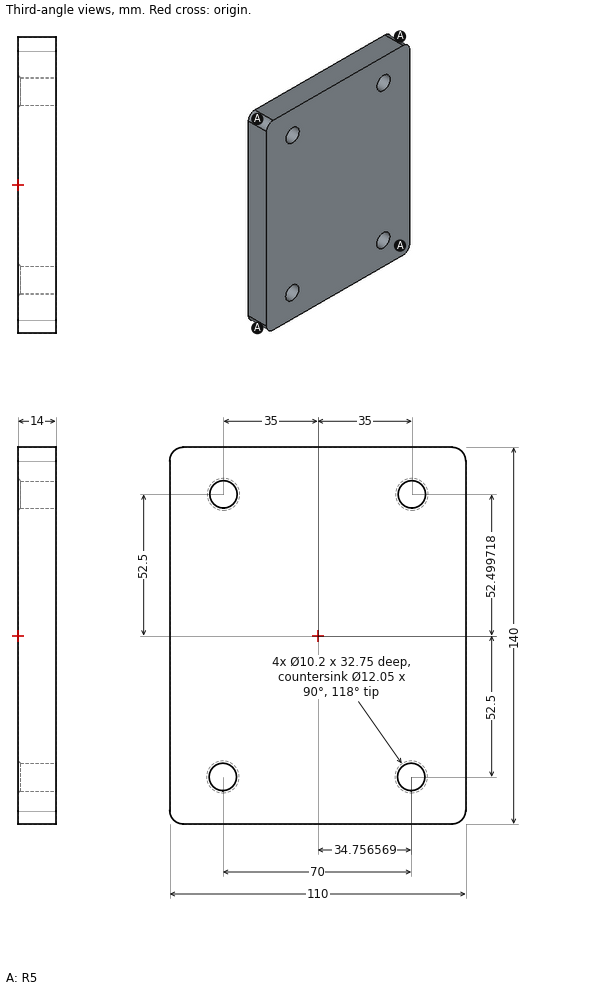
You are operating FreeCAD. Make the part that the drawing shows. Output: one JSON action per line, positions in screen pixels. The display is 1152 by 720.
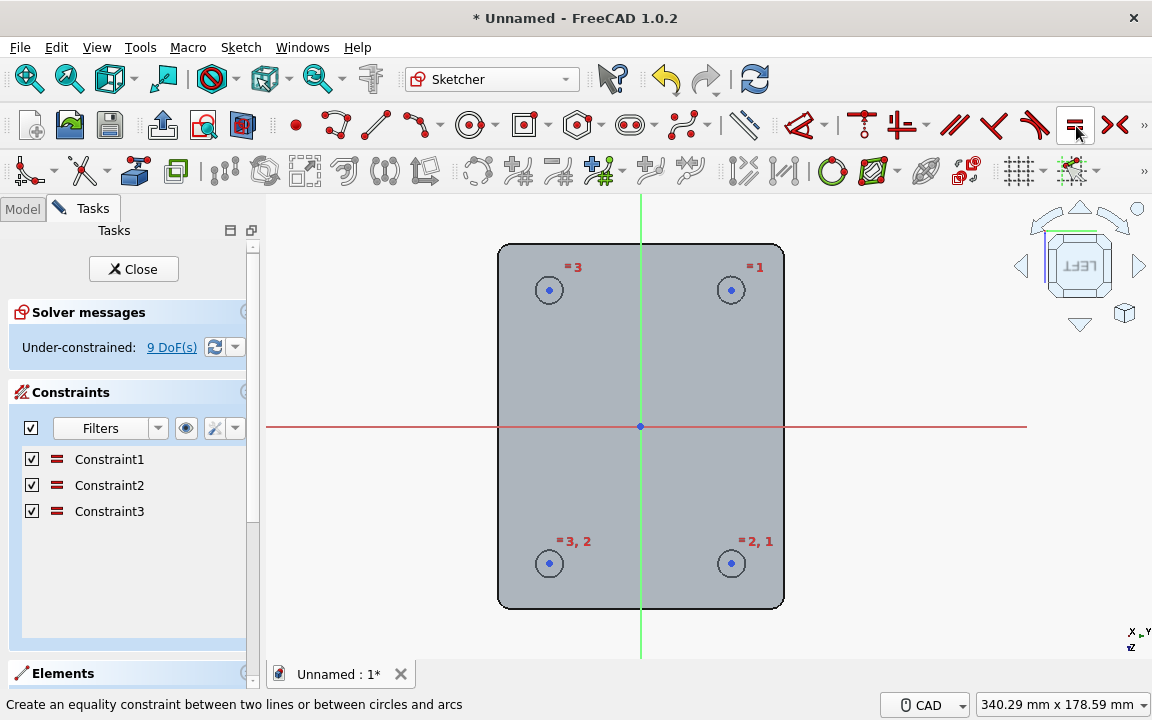
{"action": "left_click", "coordinate": [800, 126]}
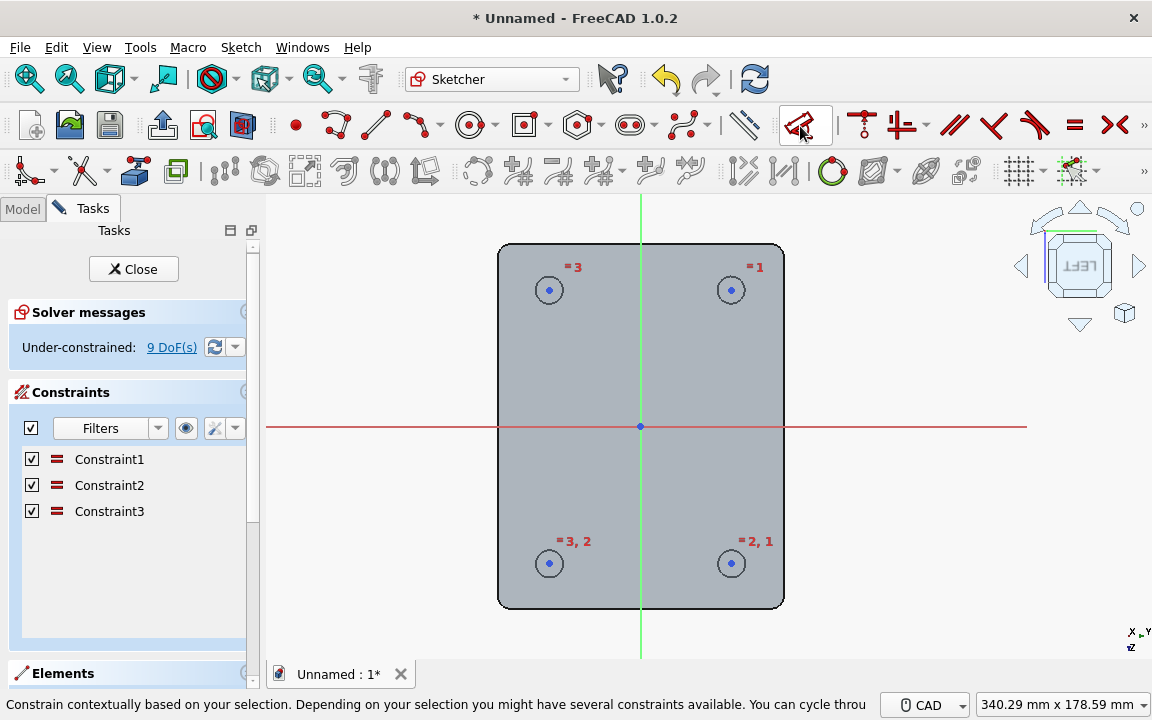
{"action": "scroll", "coordinate": [741, 280], "scroll_direction": "up", "scroll_amount": 3}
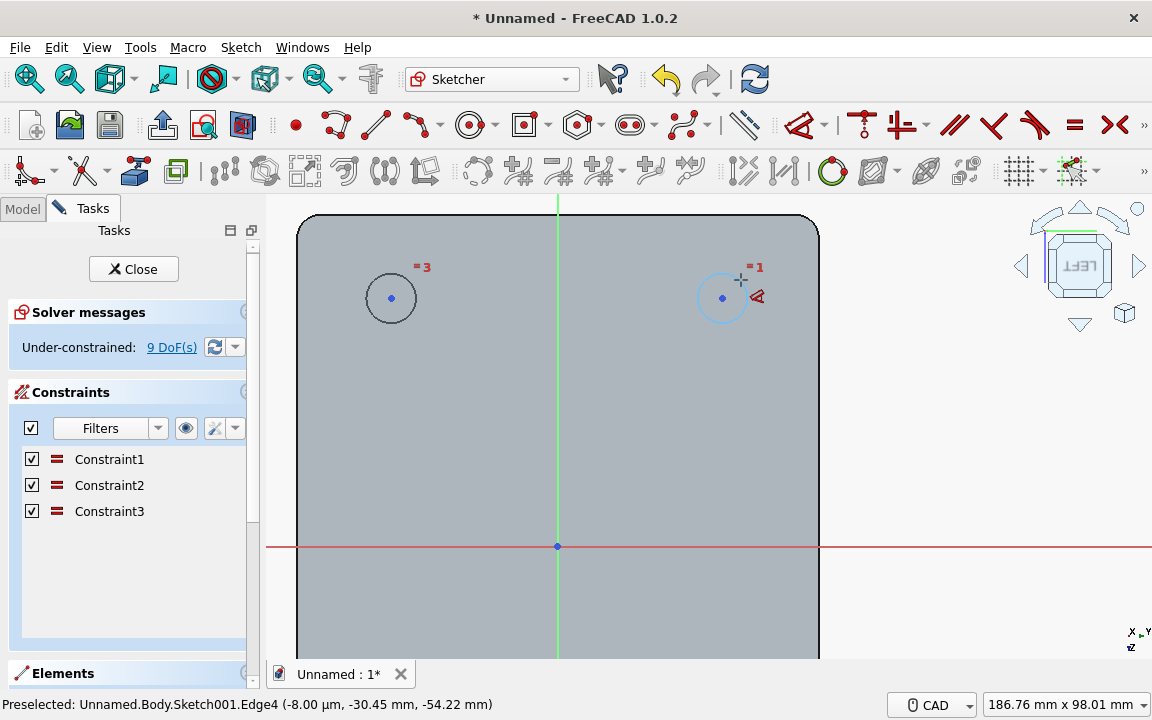
{"action": "left_click", "coordinate": [740, 281]}
{"action": "left_click", "coordinate": [763, 259]}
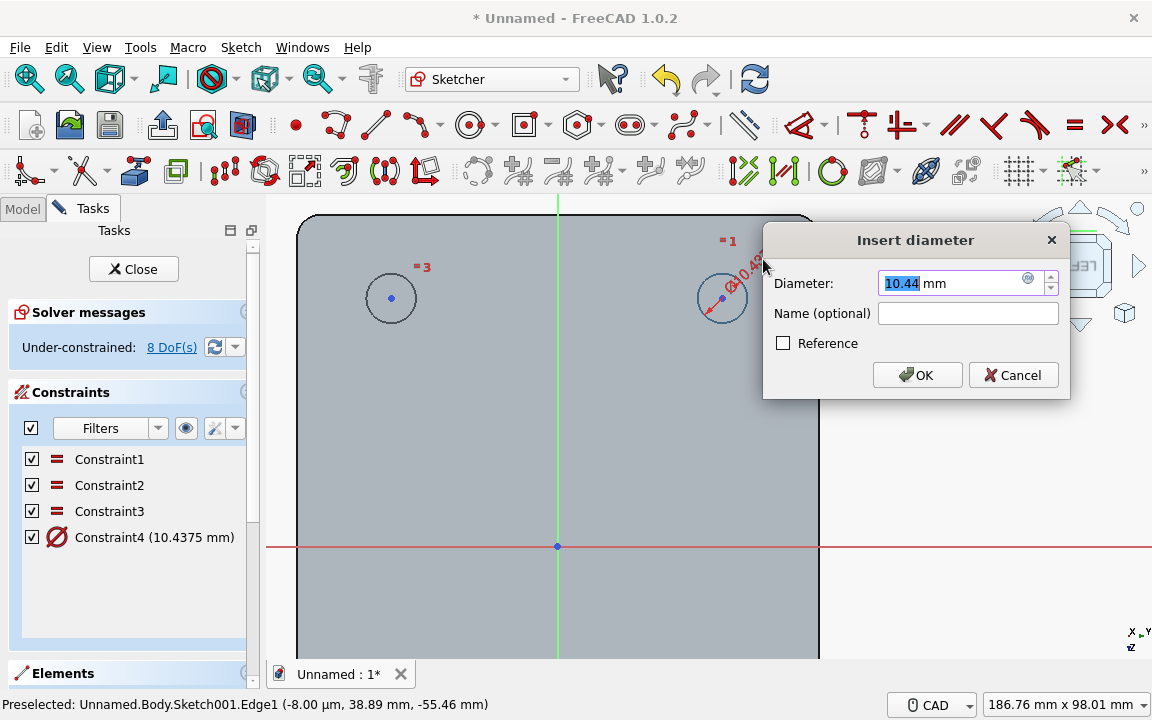
{"action": "type", "text": "10.2"}
{"action": "key", "text": "Return"}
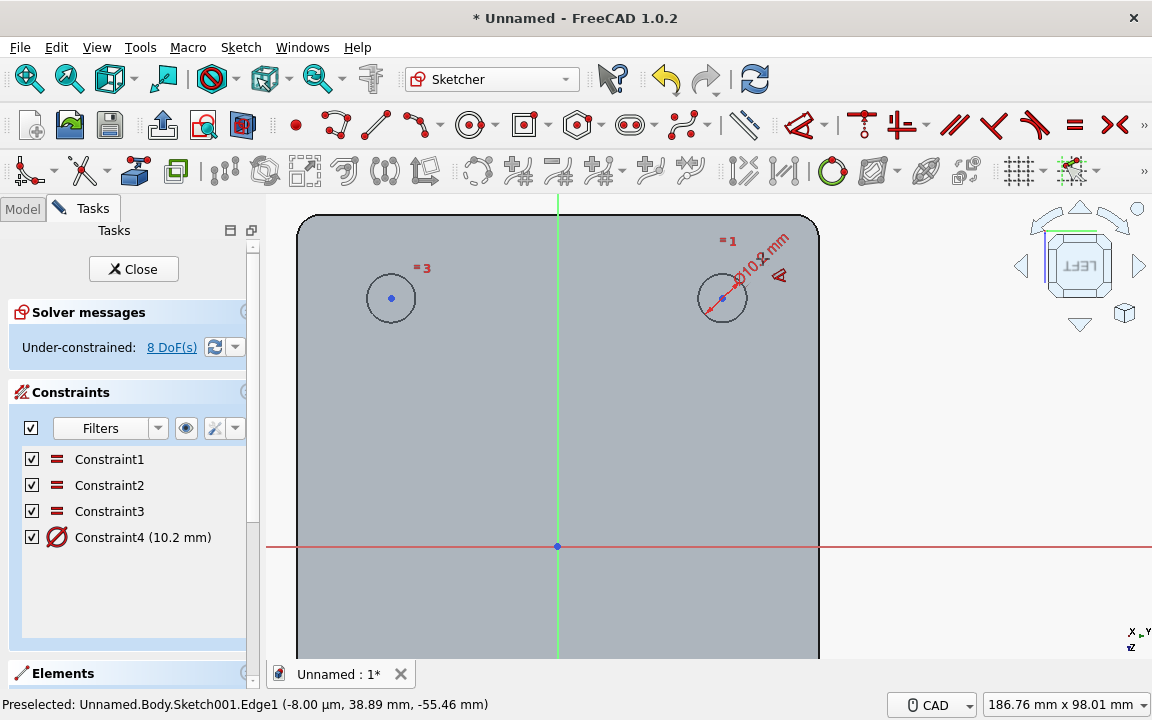
{"action": "scroll", "coordinate": [742, 280], "scroll_direction": "down", "scroll_amount": 3}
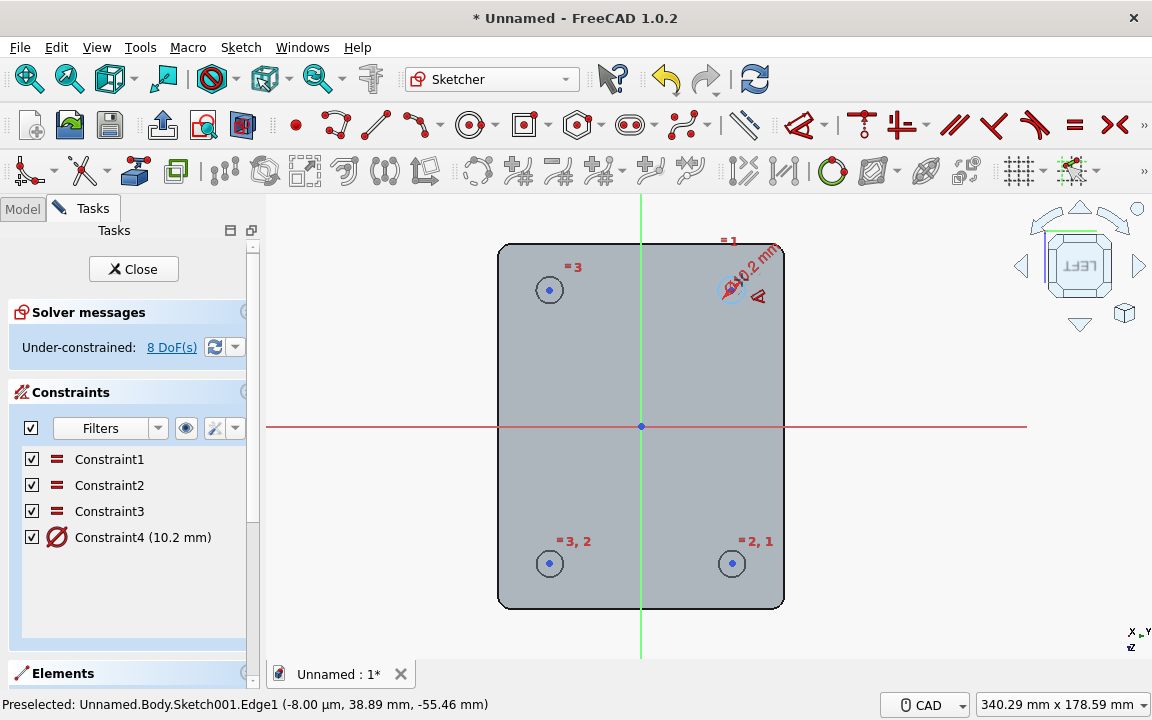
{"action": "left_click", "coordinate": [732, 564]}
{"action": "left_click", "coordinate": [687, 598]}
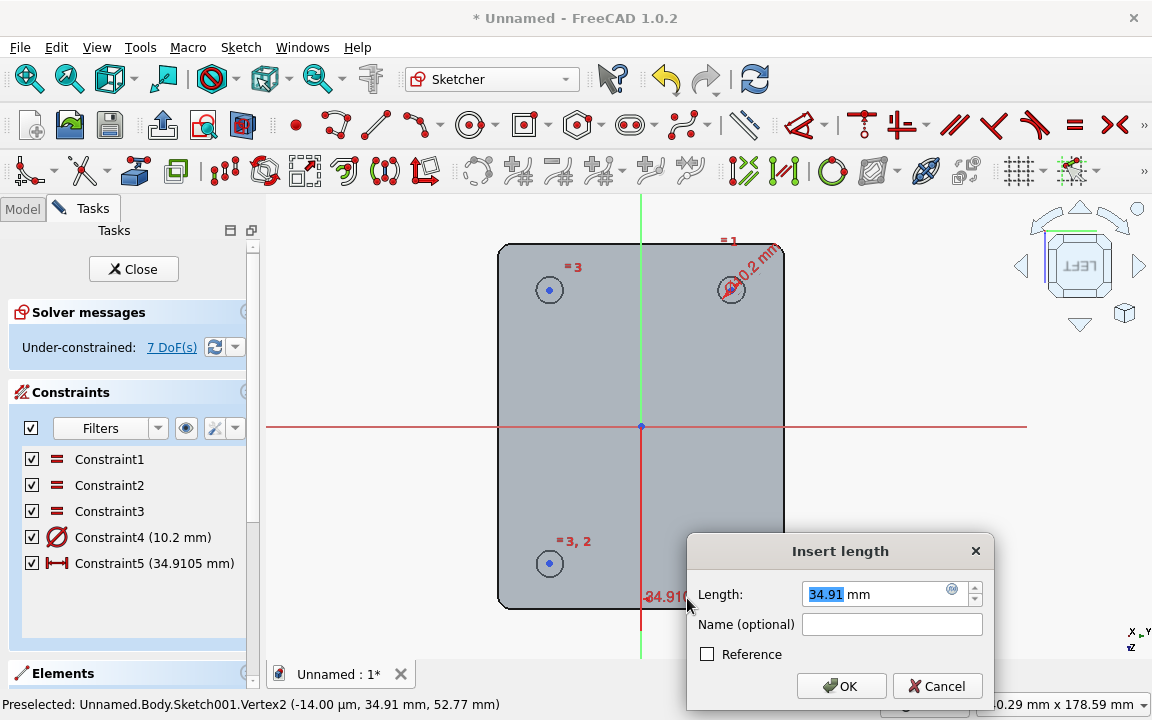
{"action": "type", "text": "35"}
{"action": "key", "text": "Return"}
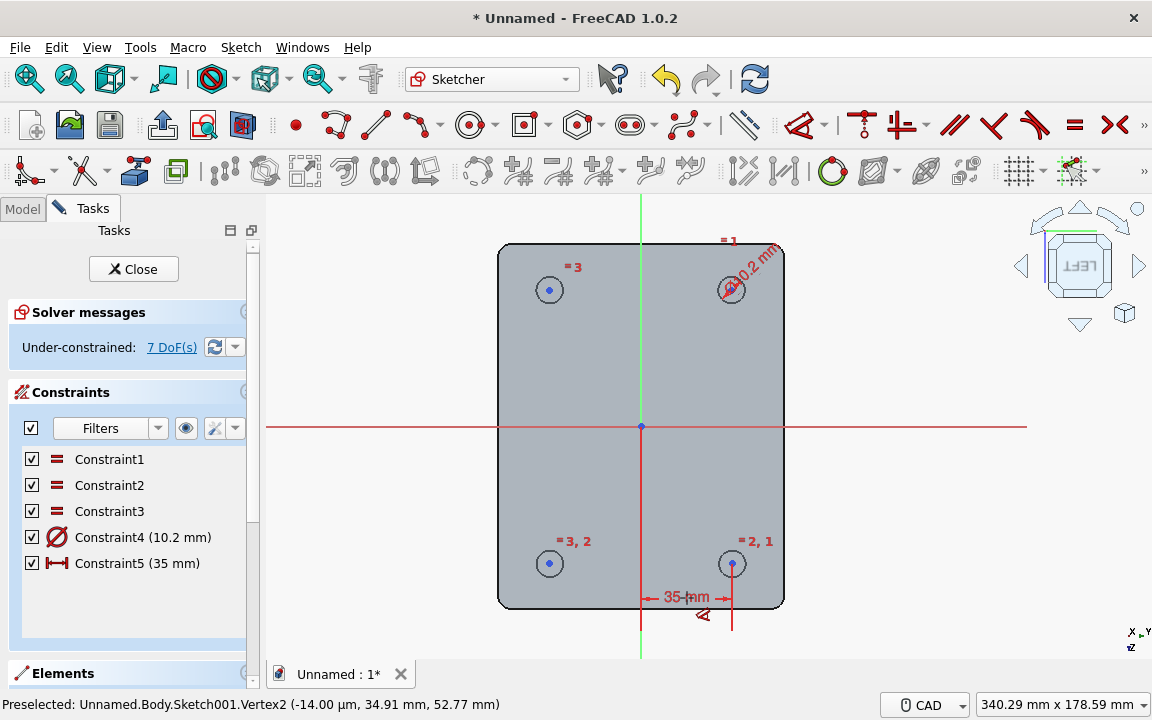
{"action": "left_click", "coordinate": [550, 564]}
{"action": "left_click", "coordinate": [596, 598]}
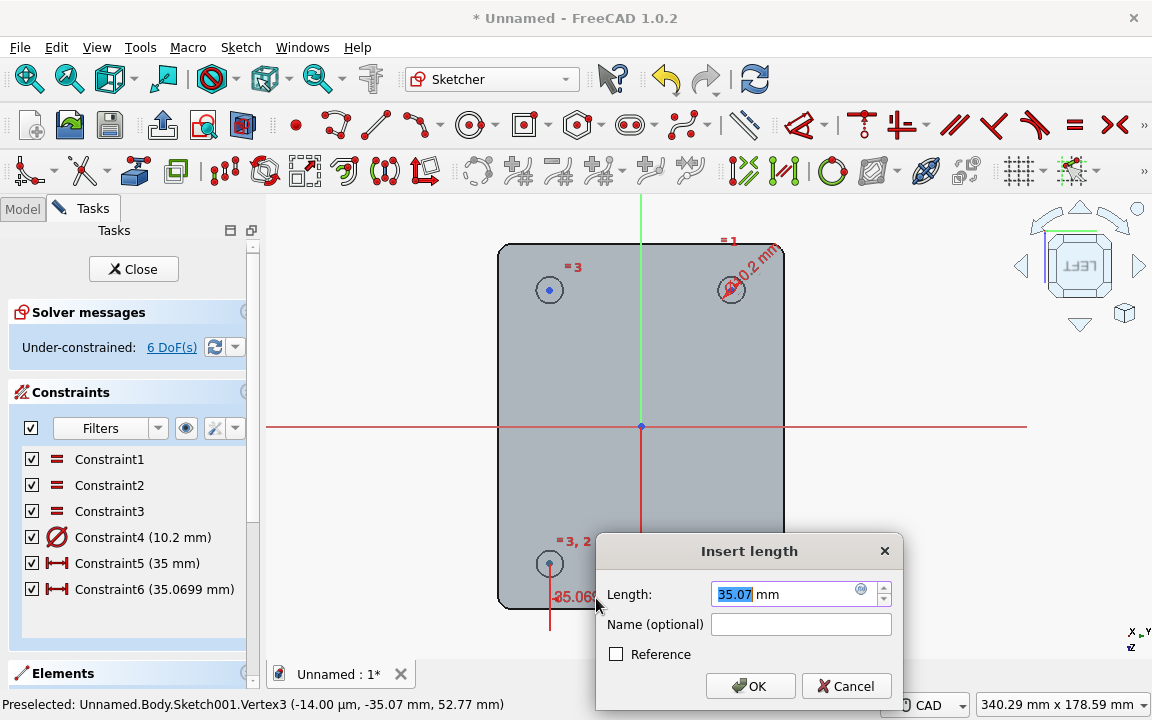
{"action": "type", "text": "35"}
{"action": "key", "text": "Return"}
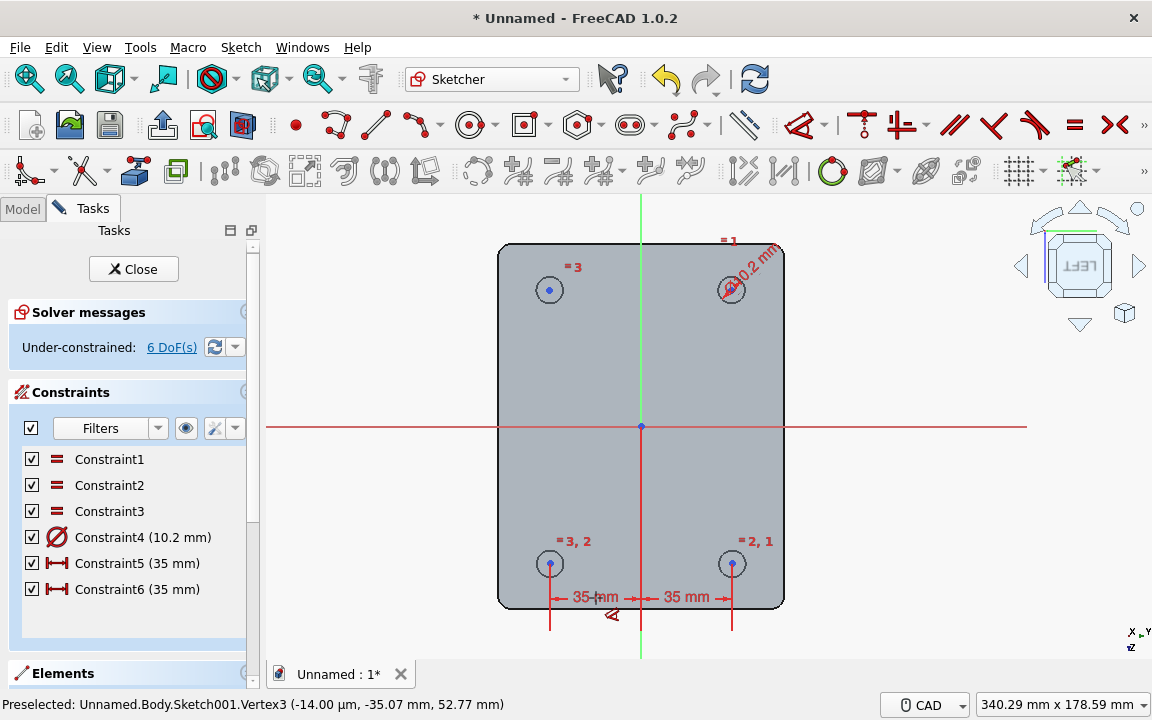
{"action": "left_click", "coordinate": [732, 290]}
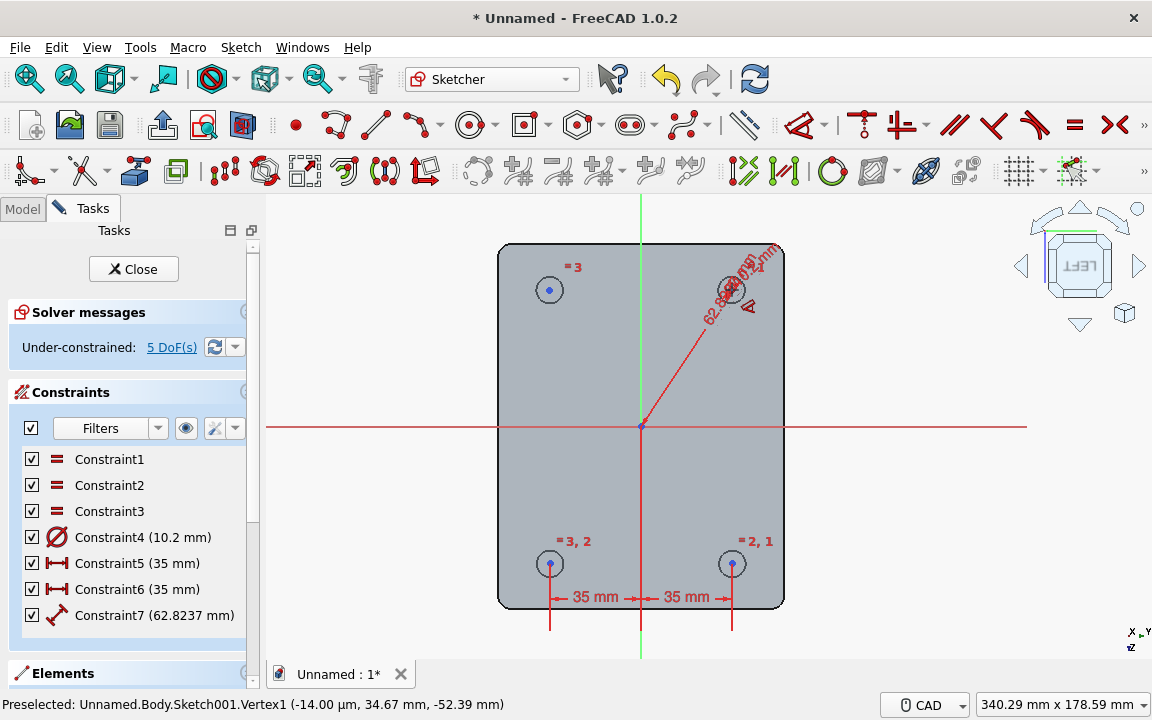
{"action": "left_click", "coordinate": [550, 290]}
{"action": "left_click", "coordinate": [599, 256]}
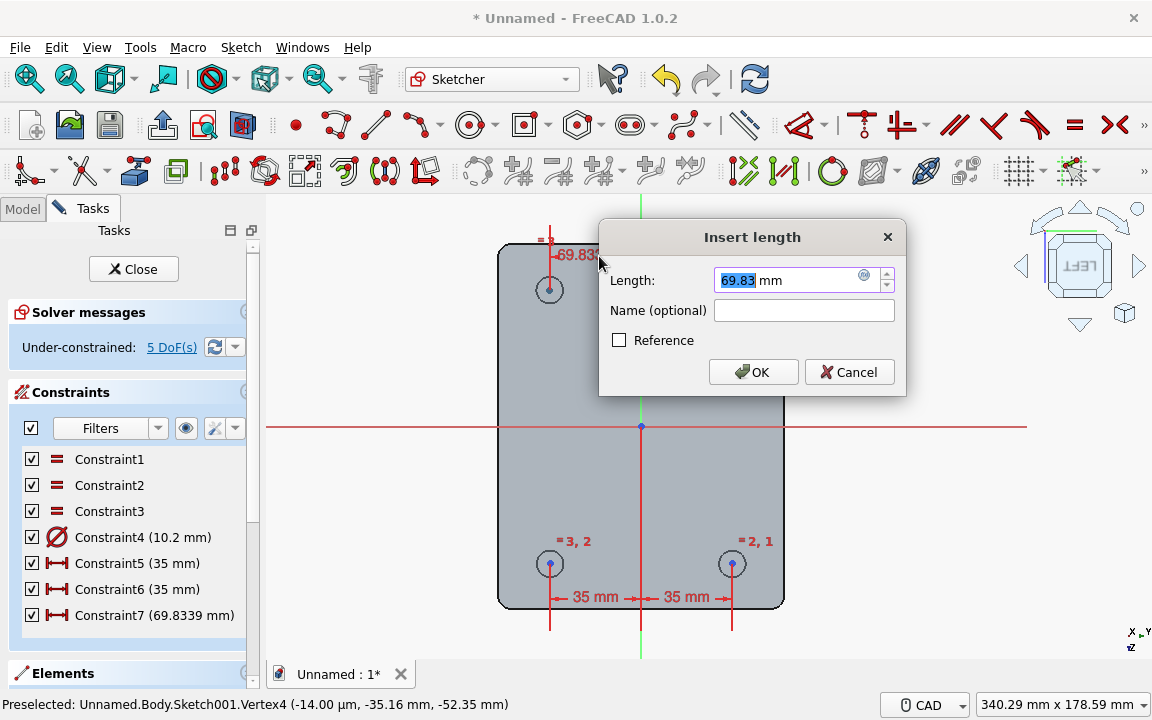
{"action": "type", "text": "70"}
{"action": "key", "text": "Return"}